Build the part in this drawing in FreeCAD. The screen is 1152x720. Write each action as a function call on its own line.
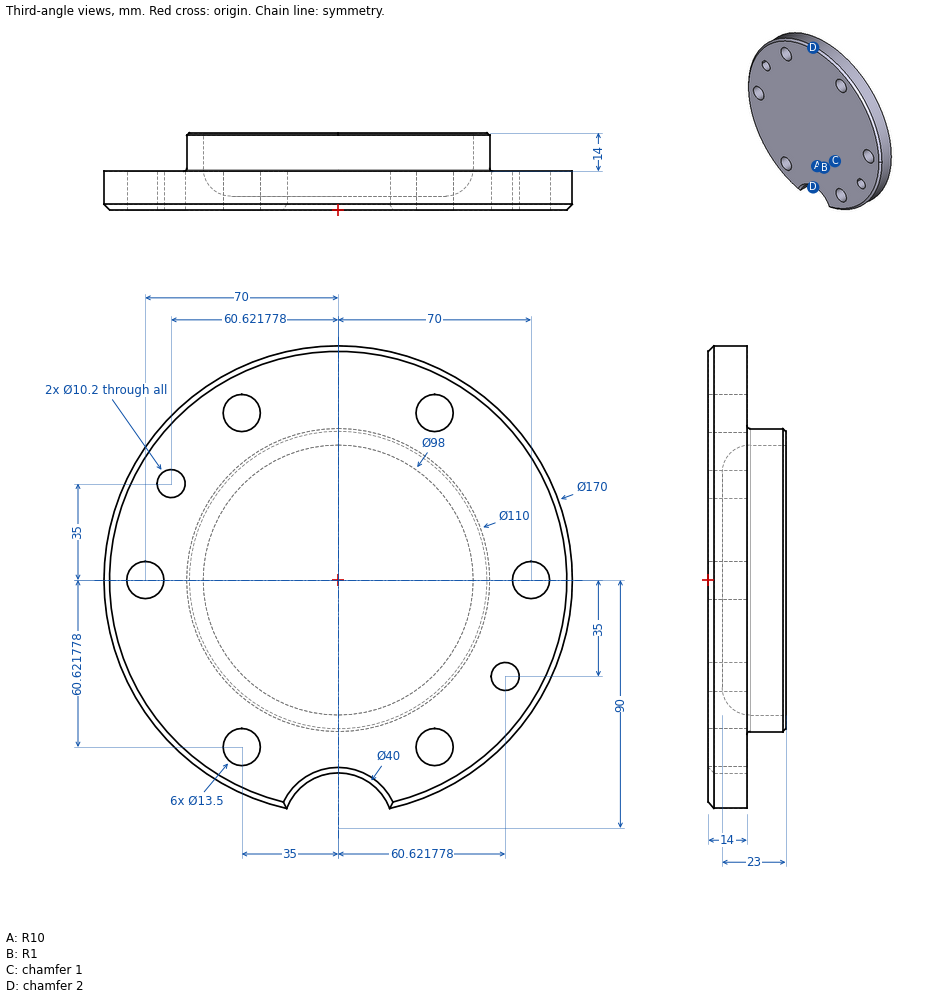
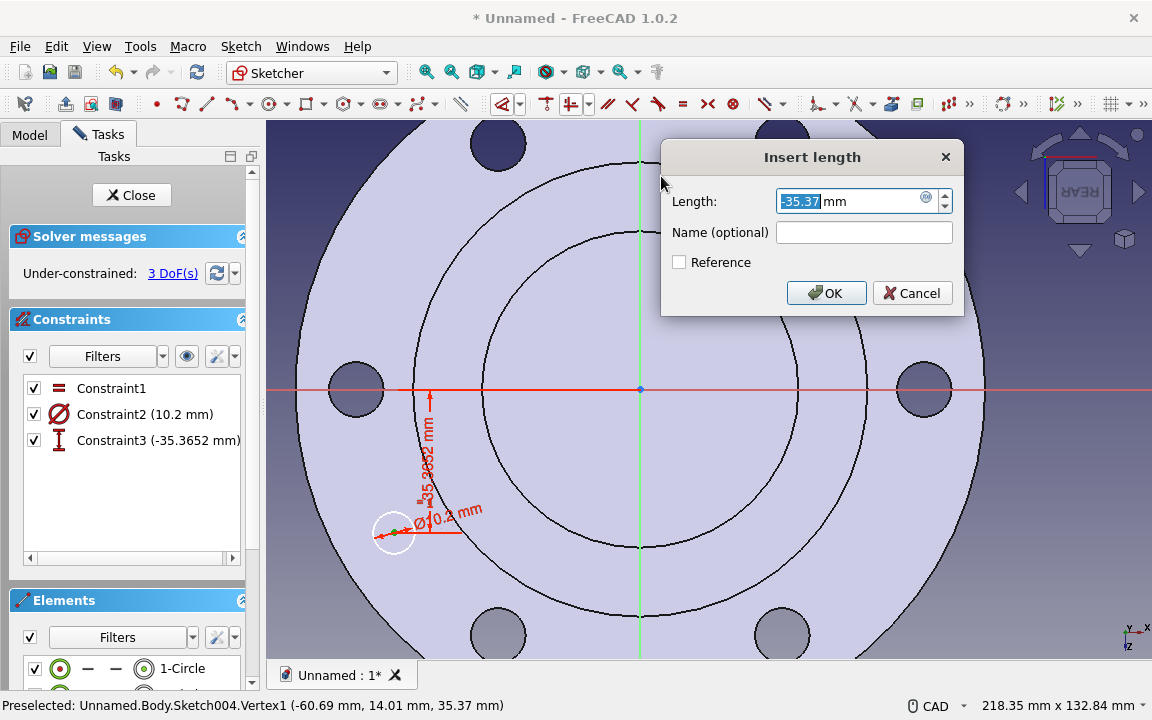
text(-35)
key(Return)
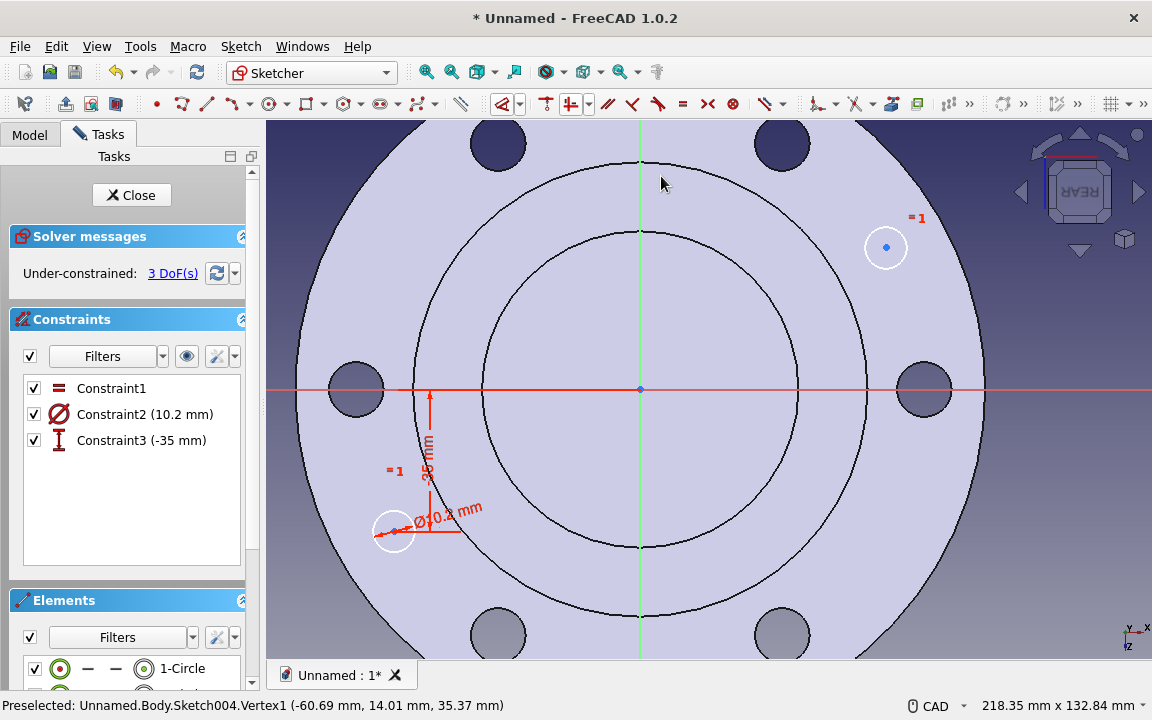
click(886, 248)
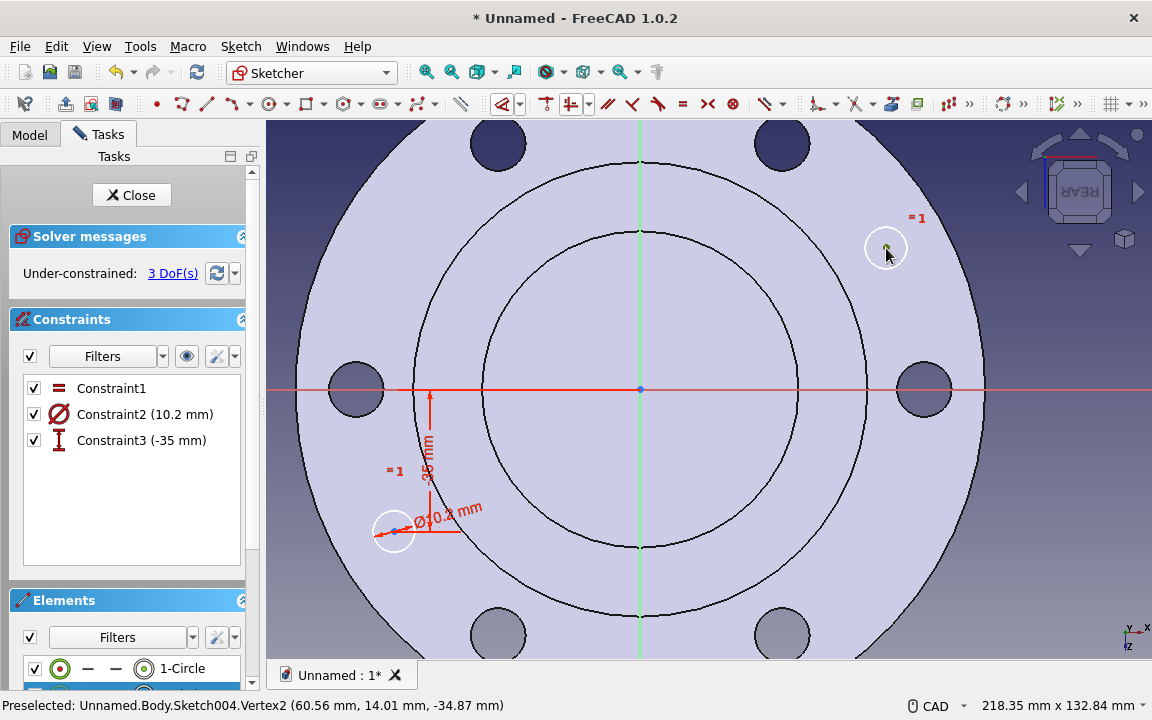
key(i)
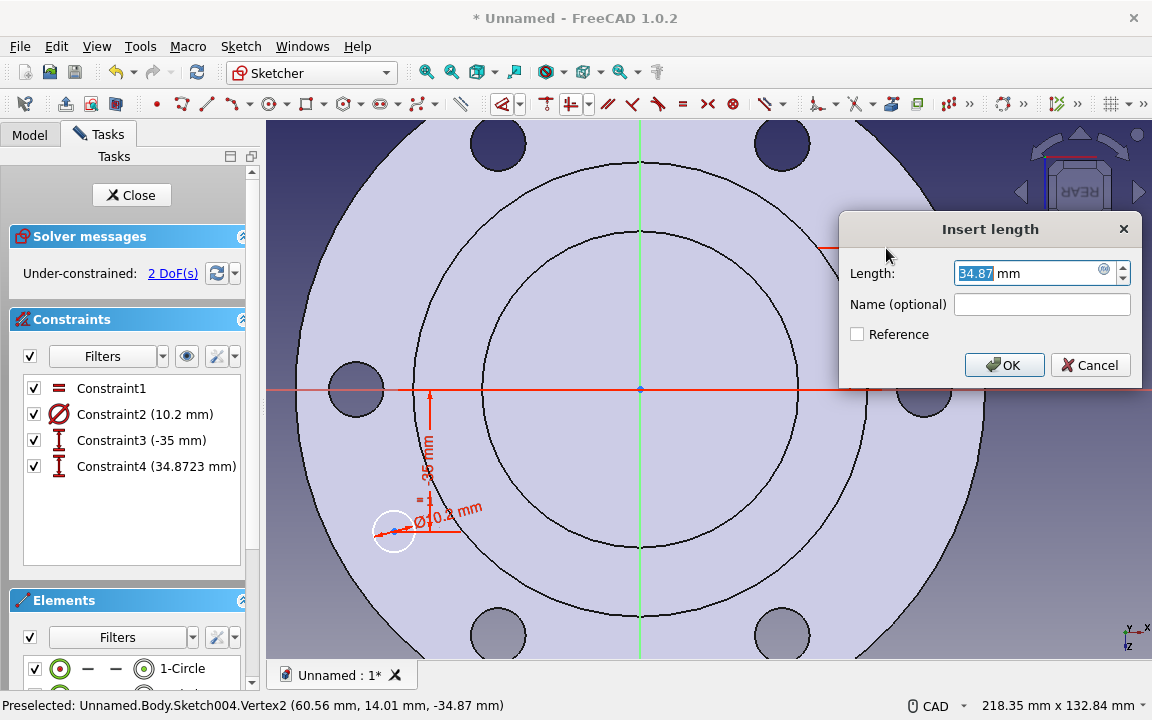
text(35)
key(Return)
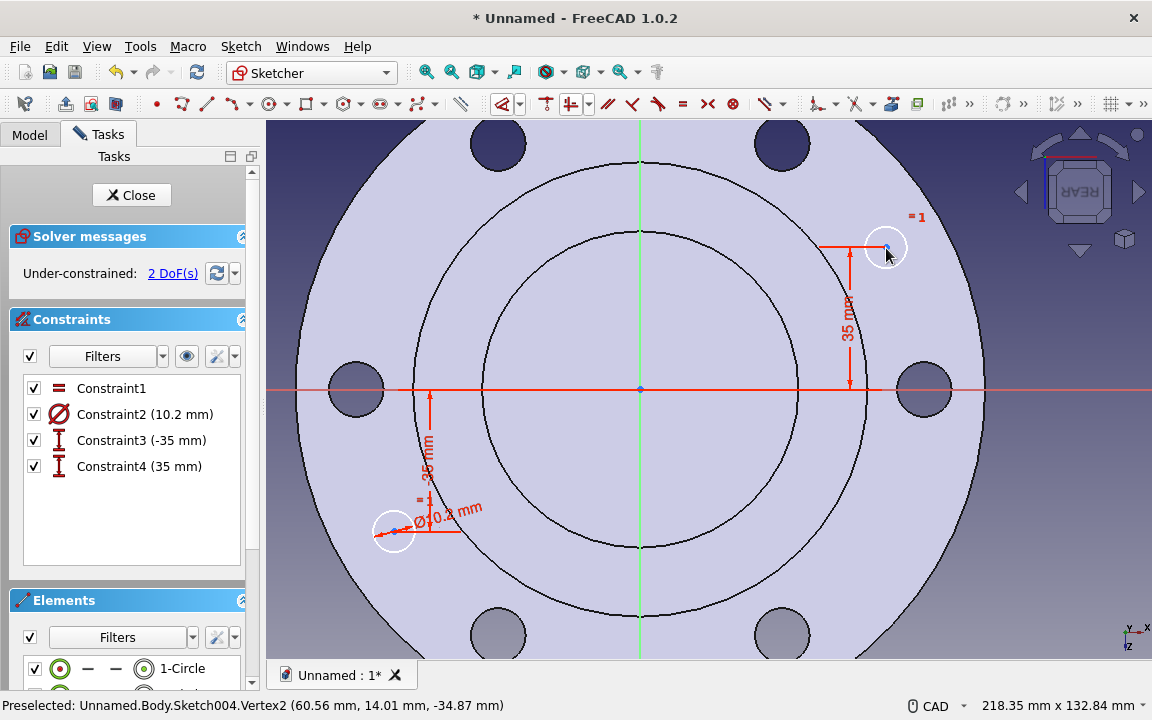
click(394, 532)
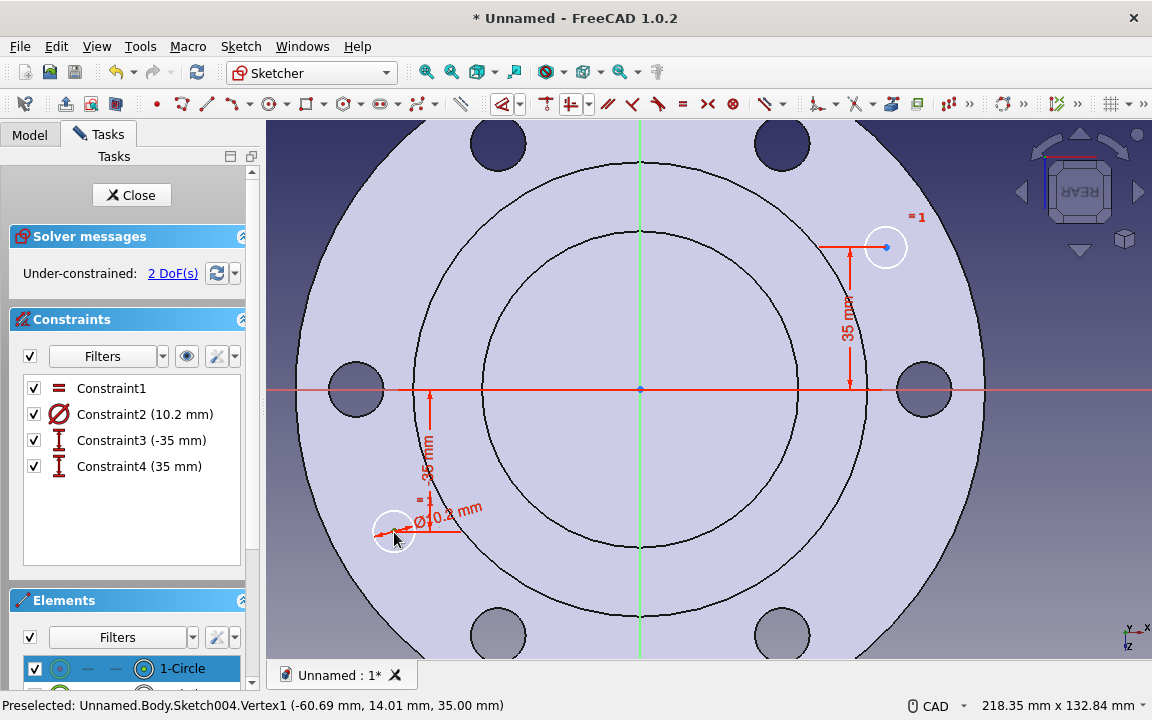
click(520, 104)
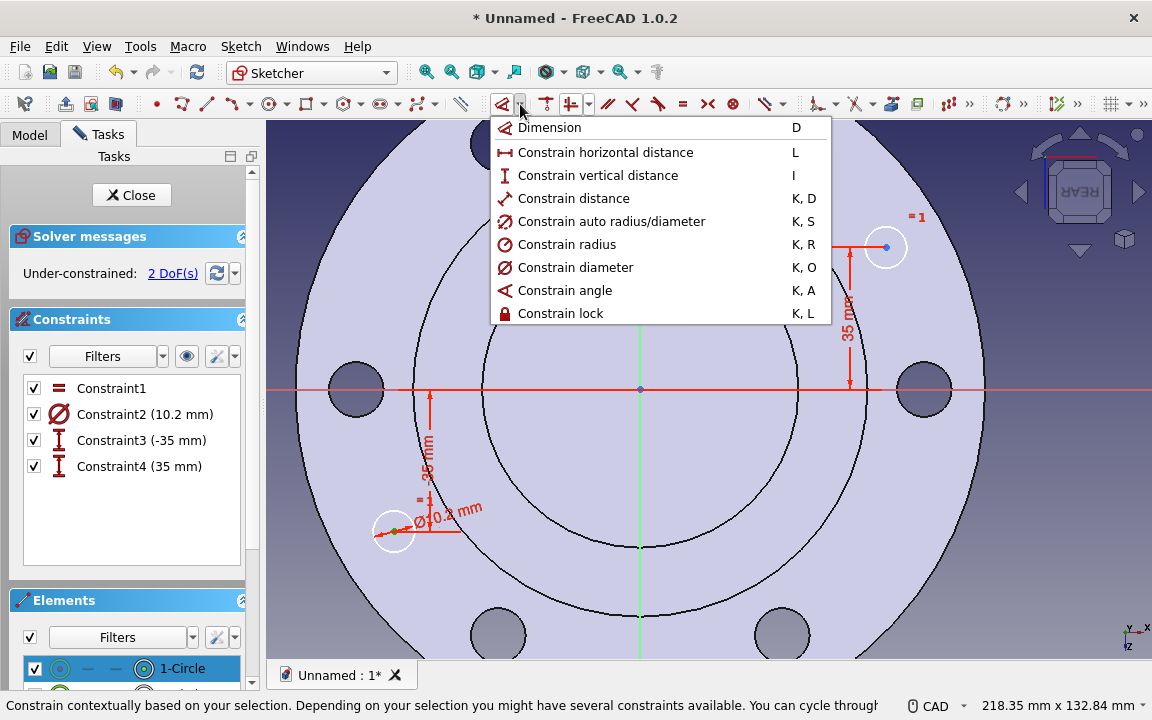
click(661, 152)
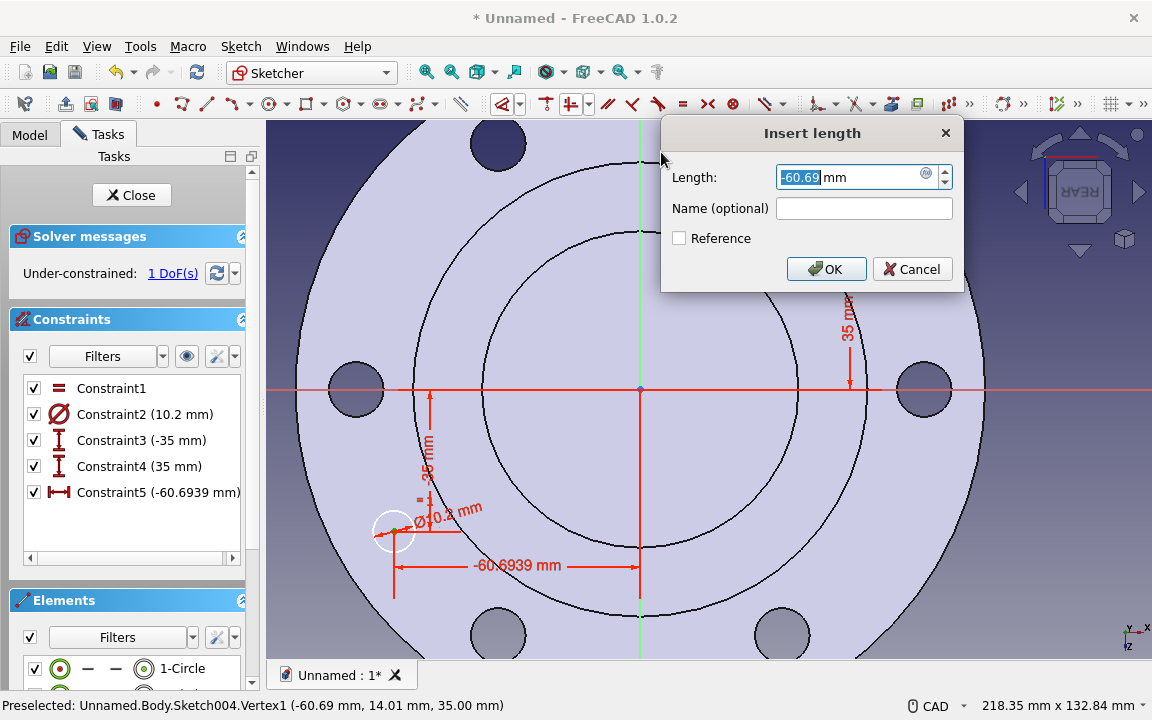
text(-60.621778)
key(Return)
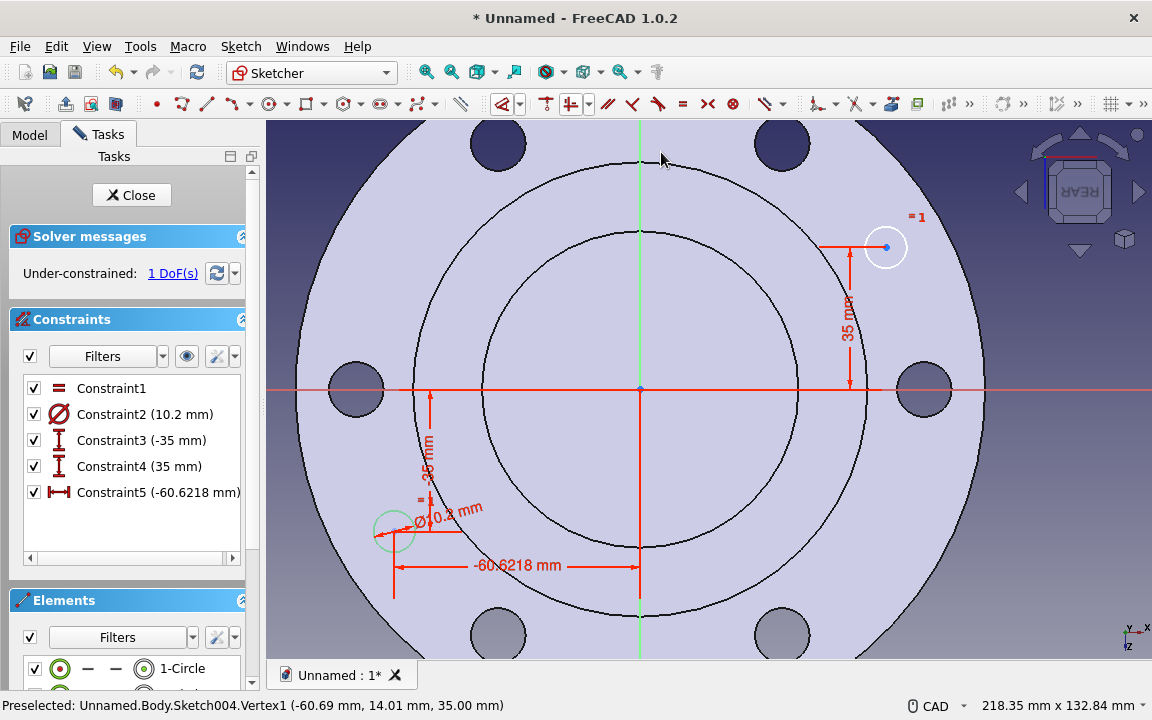
click(886, 247)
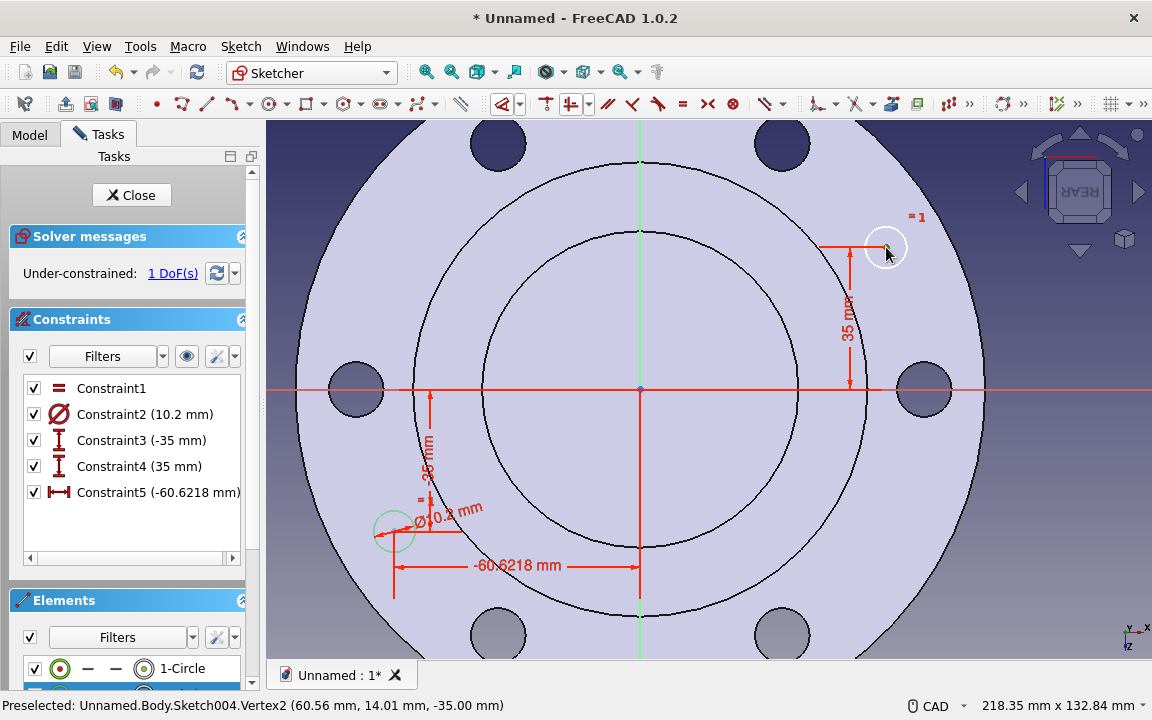
key(l)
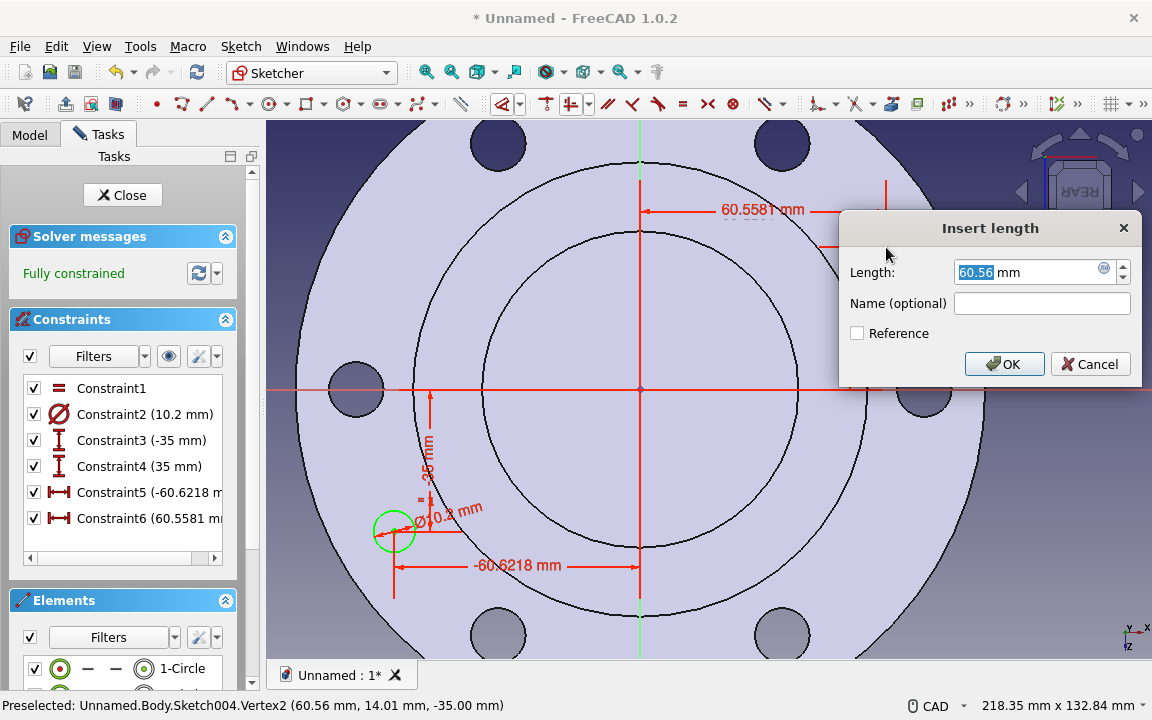
text(60.621778)
key(Return)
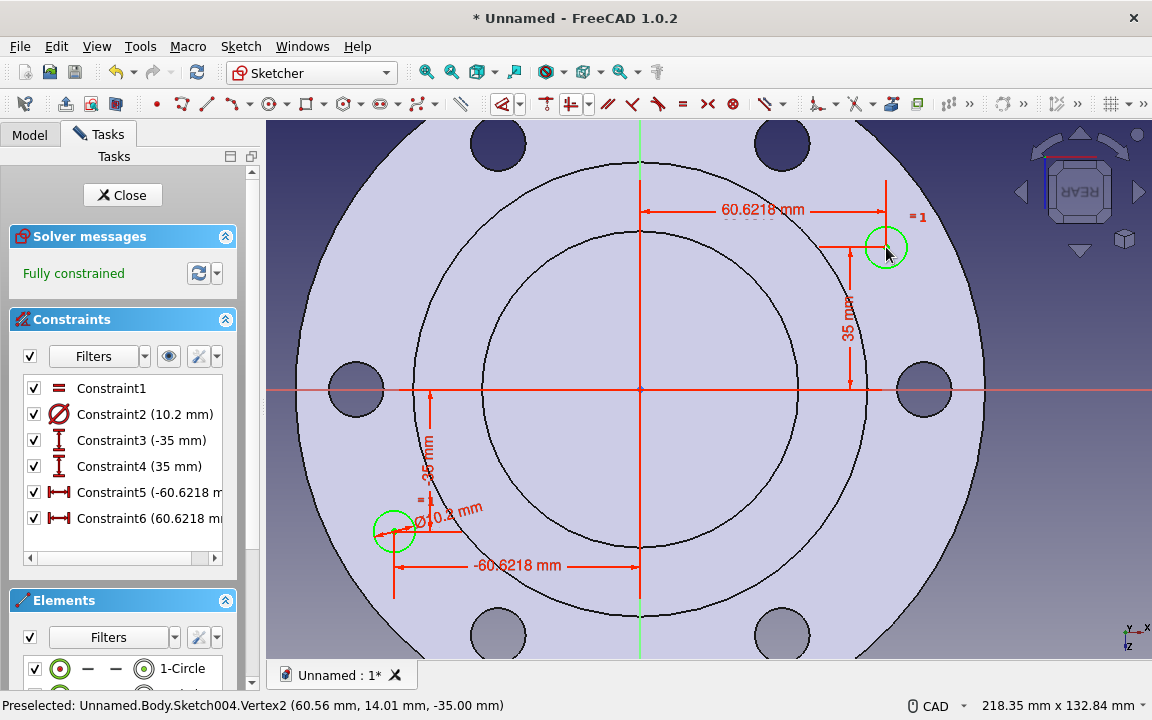
click(123, 195)